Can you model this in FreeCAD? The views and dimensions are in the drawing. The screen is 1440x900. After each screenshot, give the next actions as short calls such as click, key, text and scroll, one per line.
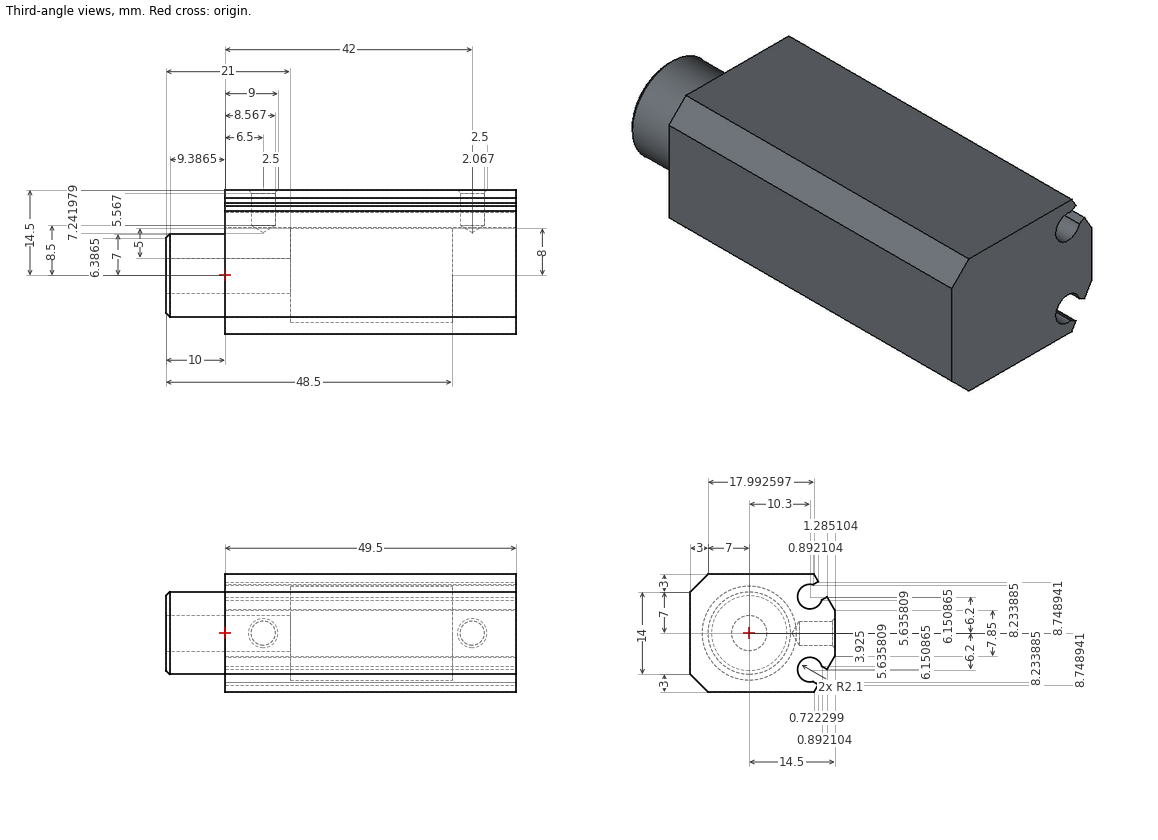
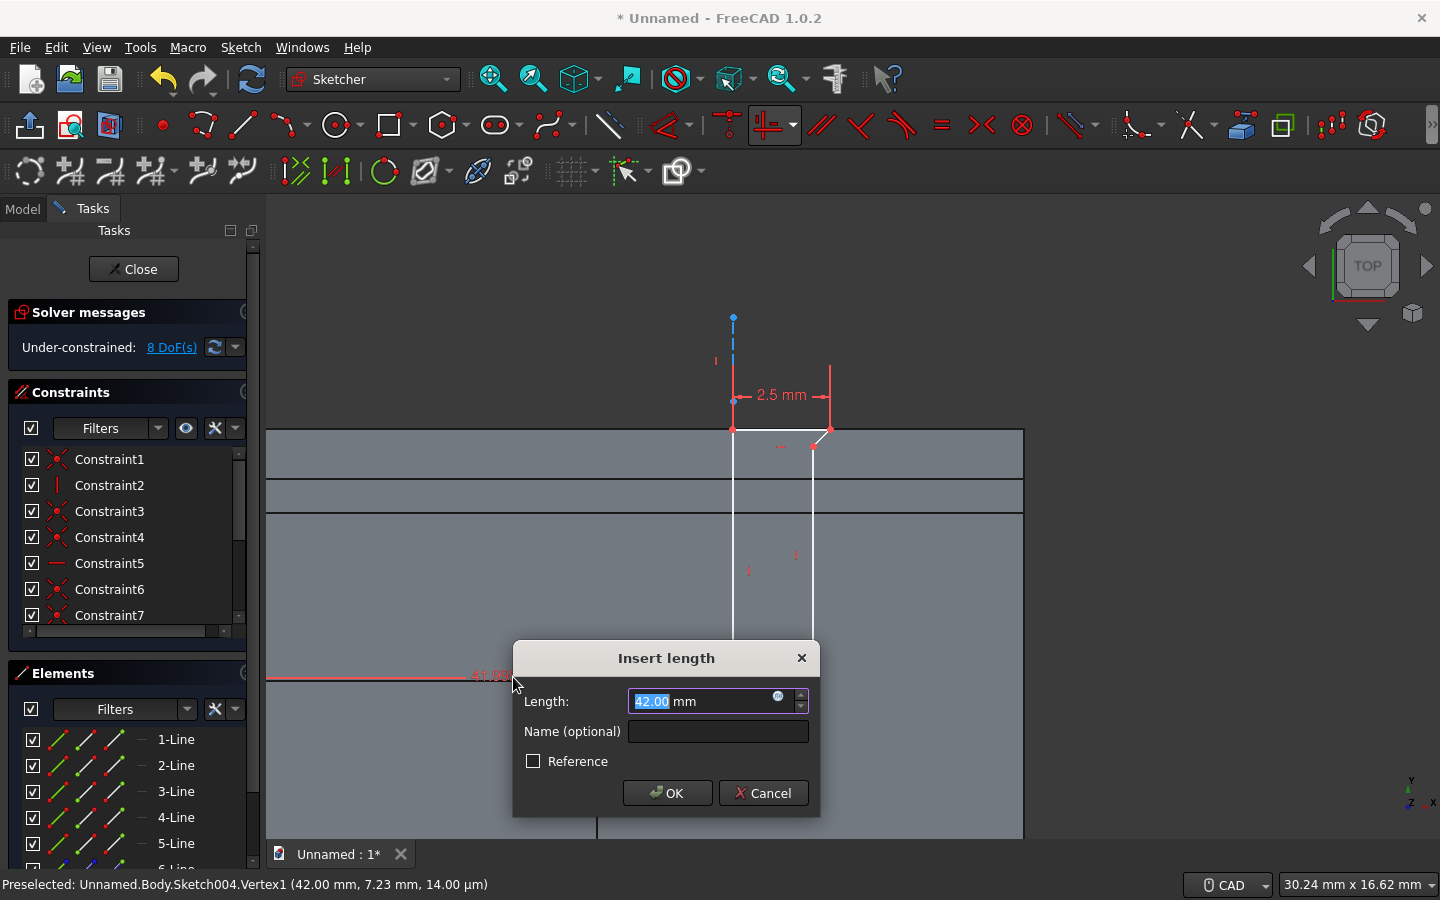
text(42)
key(Return)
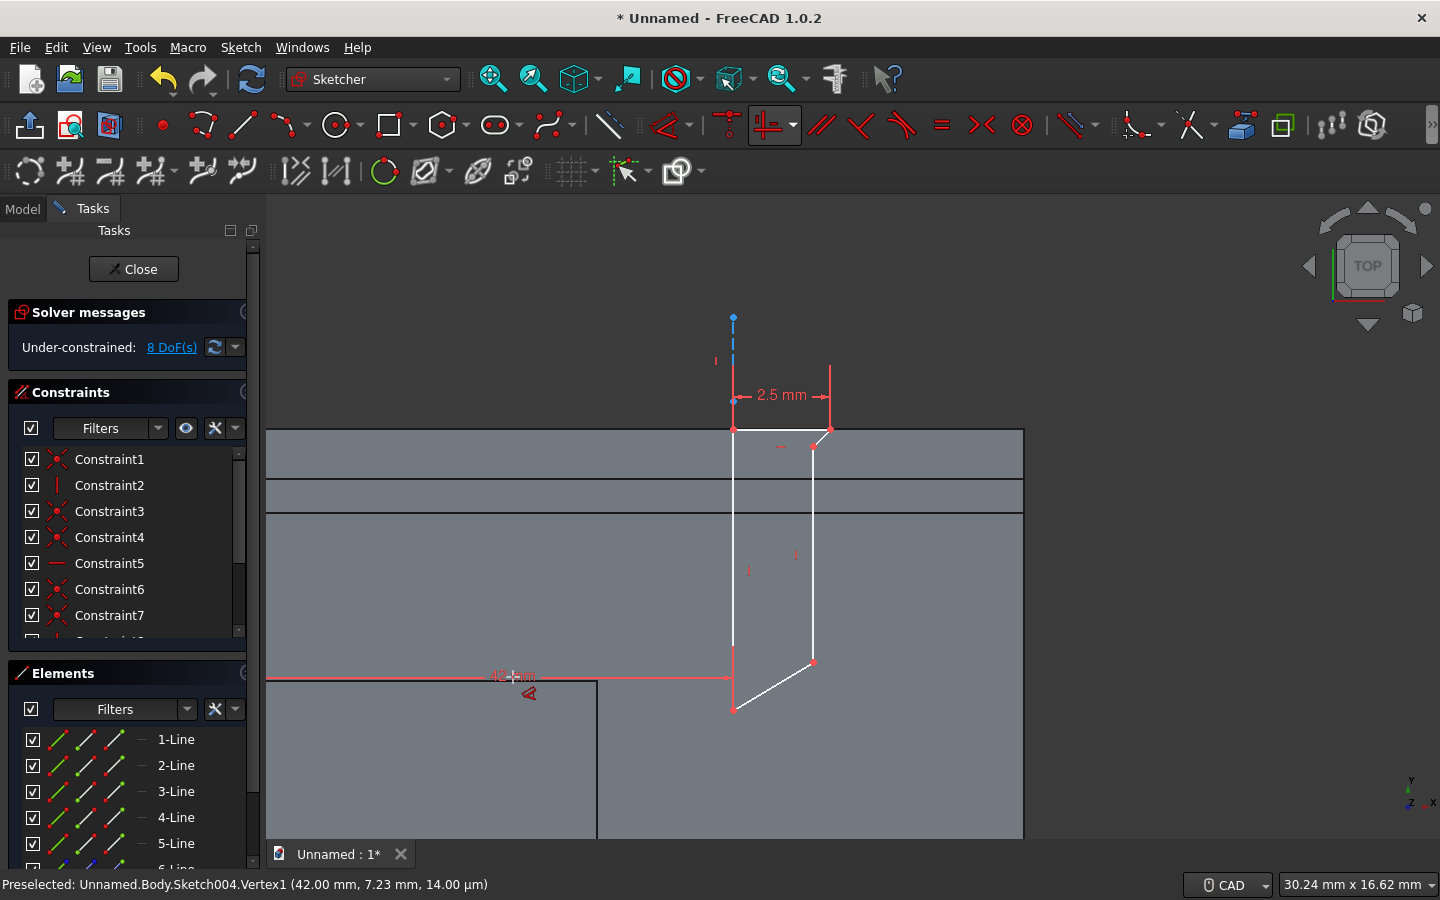
click(733, 402)
click(514, 368)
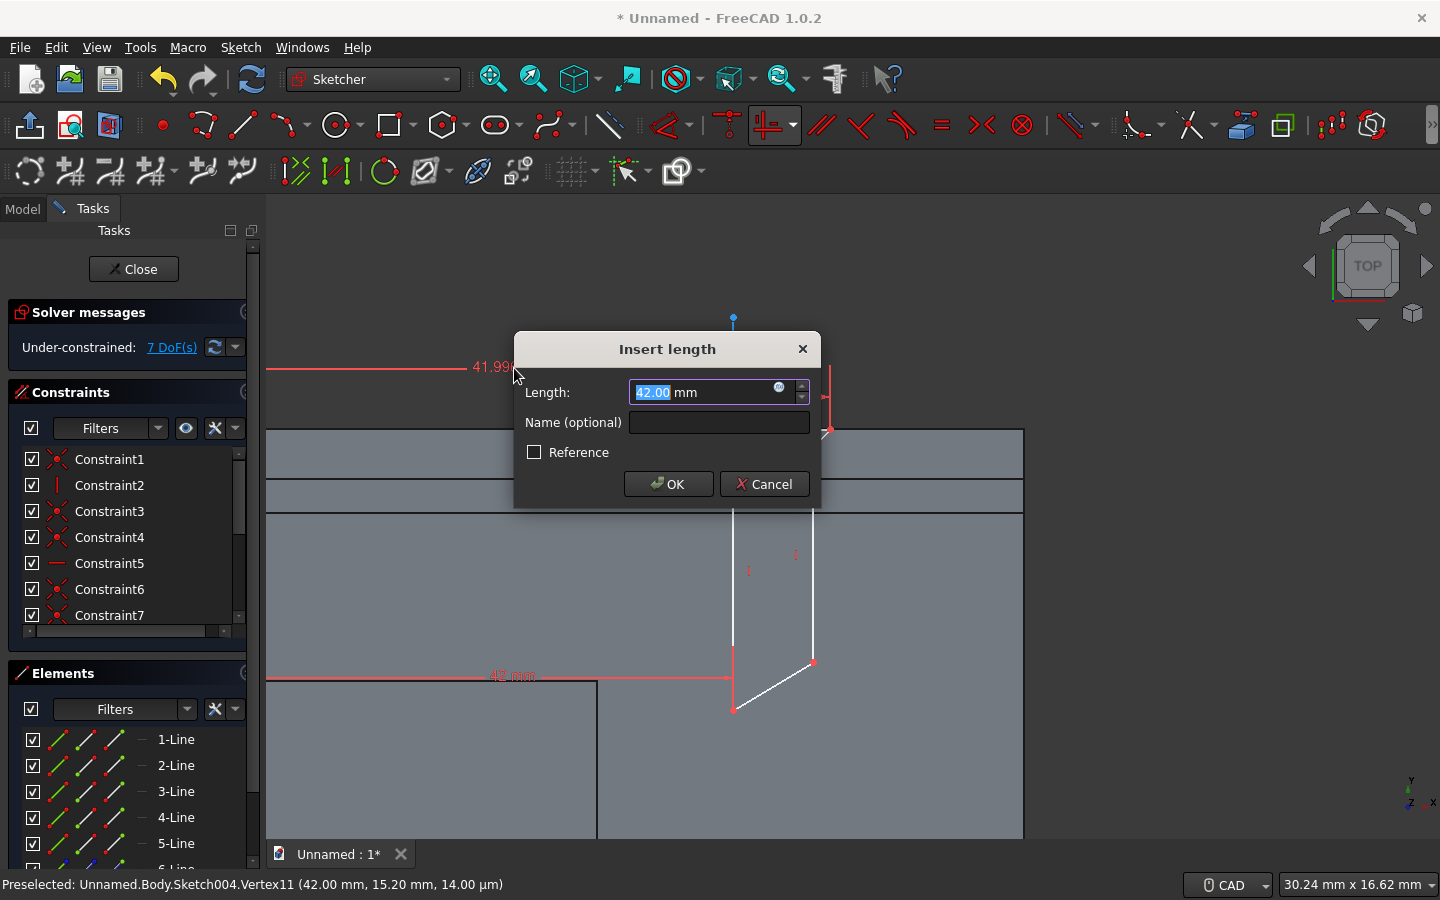
text(42)
key(Return)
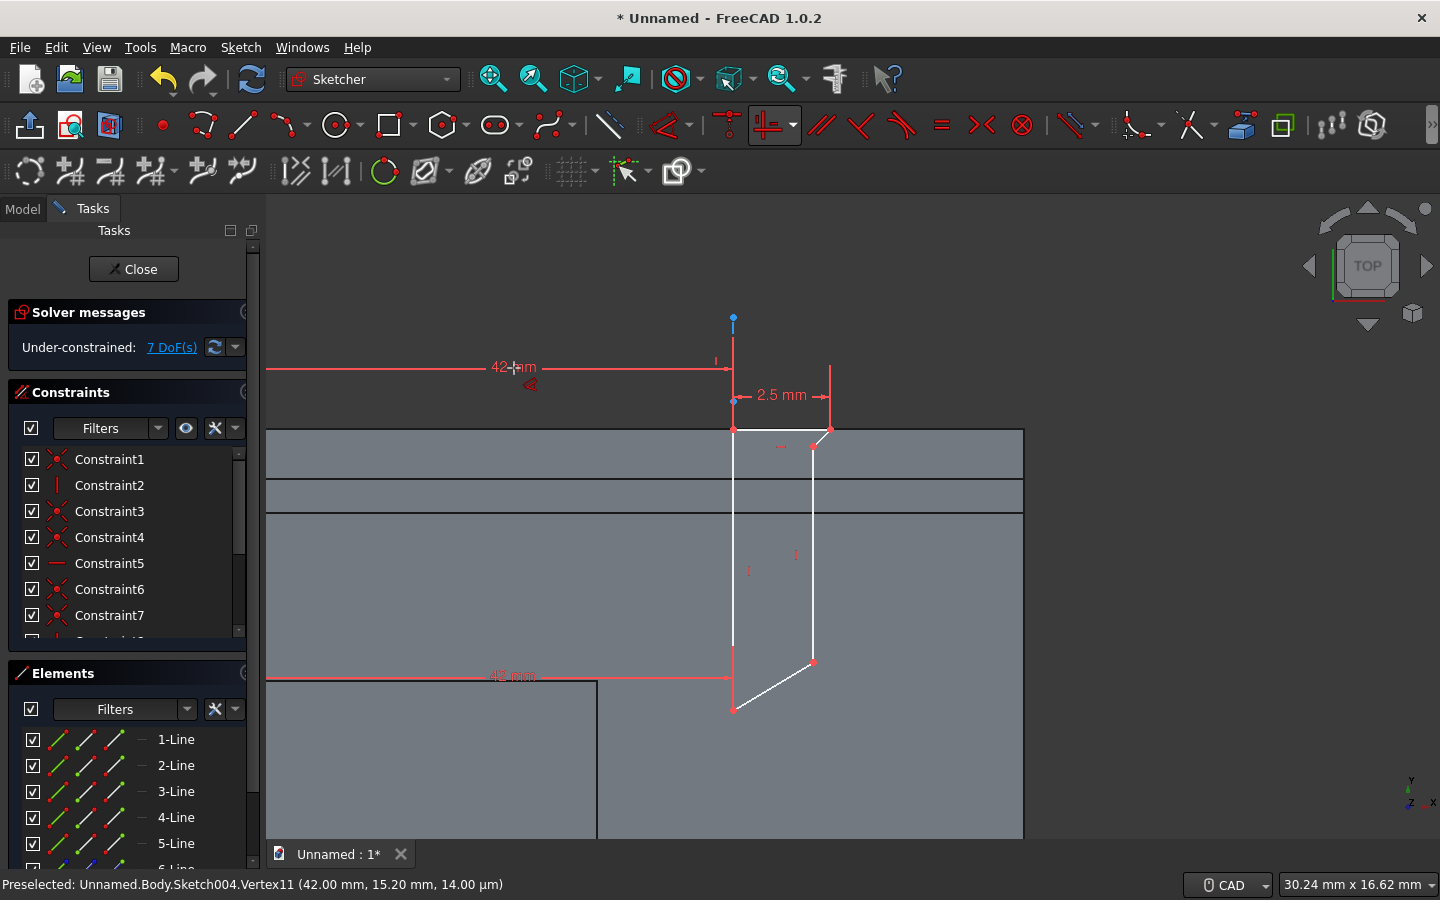
click(813, 663)
click(847, 737)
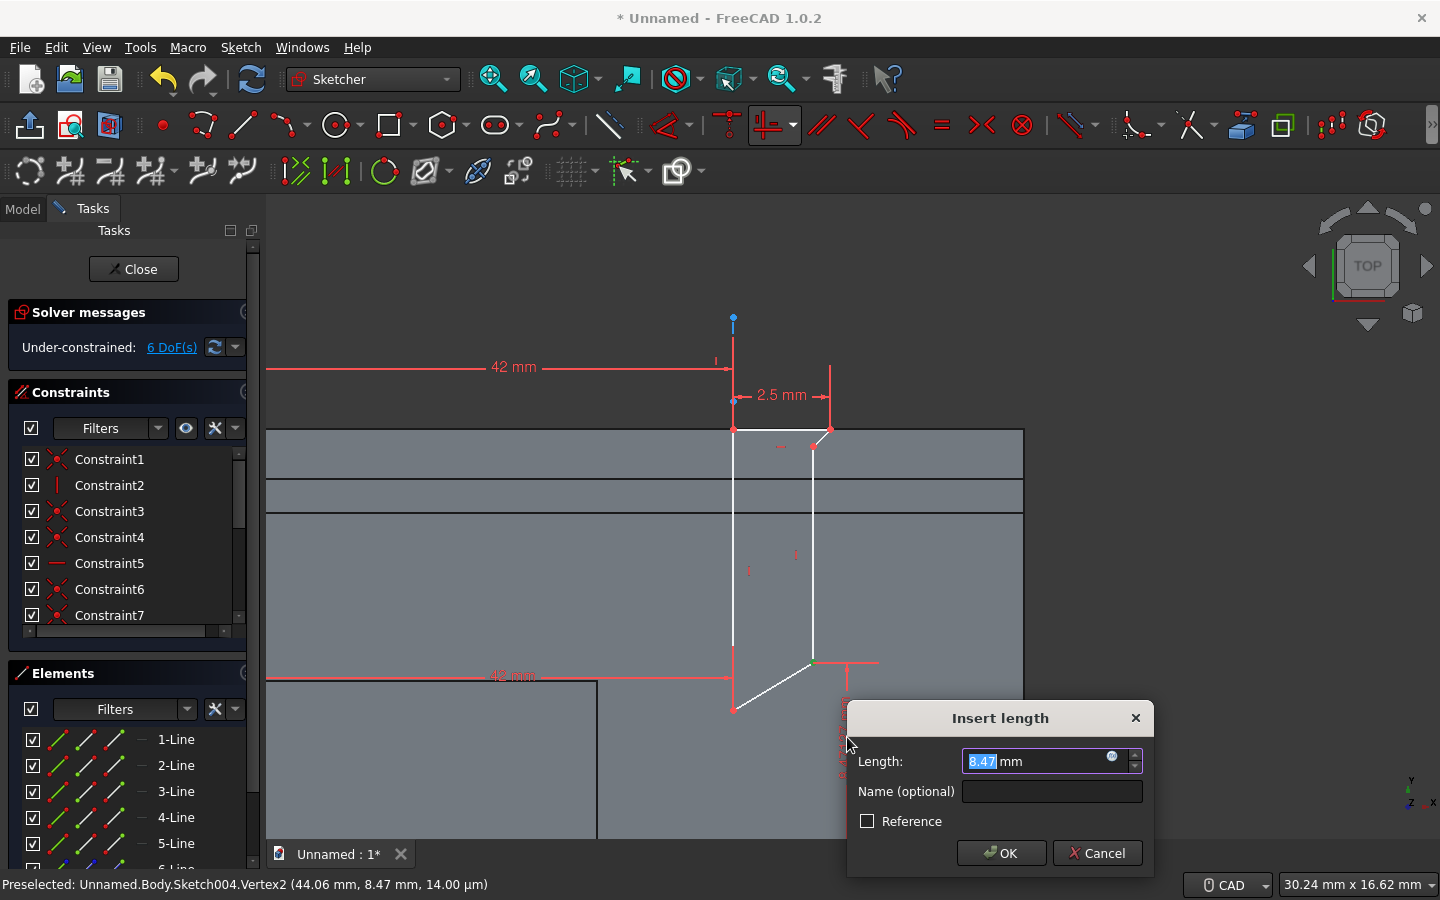
text(8.5)
key(Return)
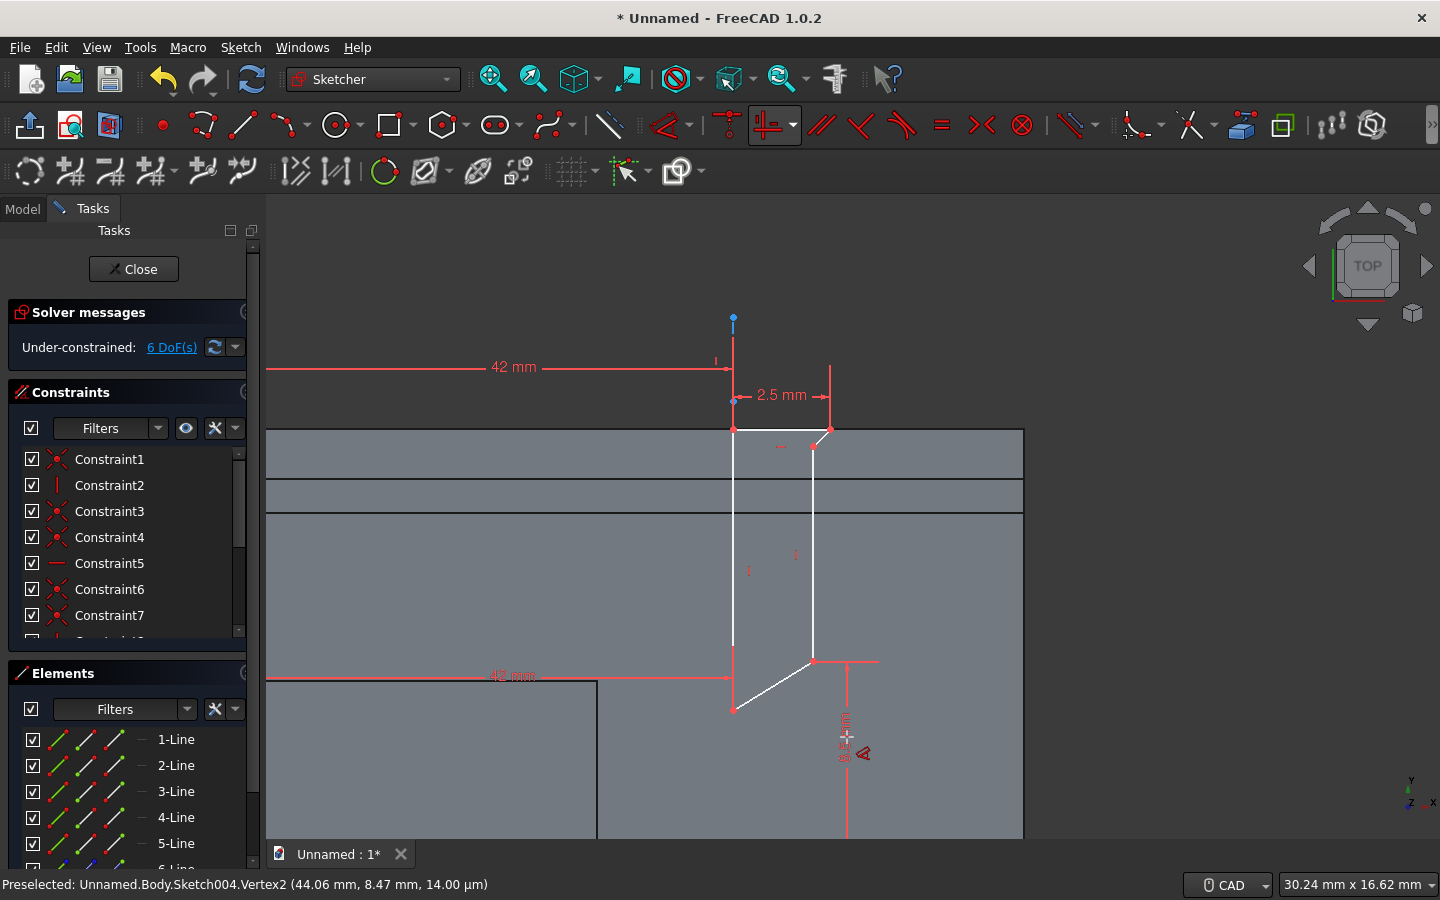
click(813, 597)
click(847, 554)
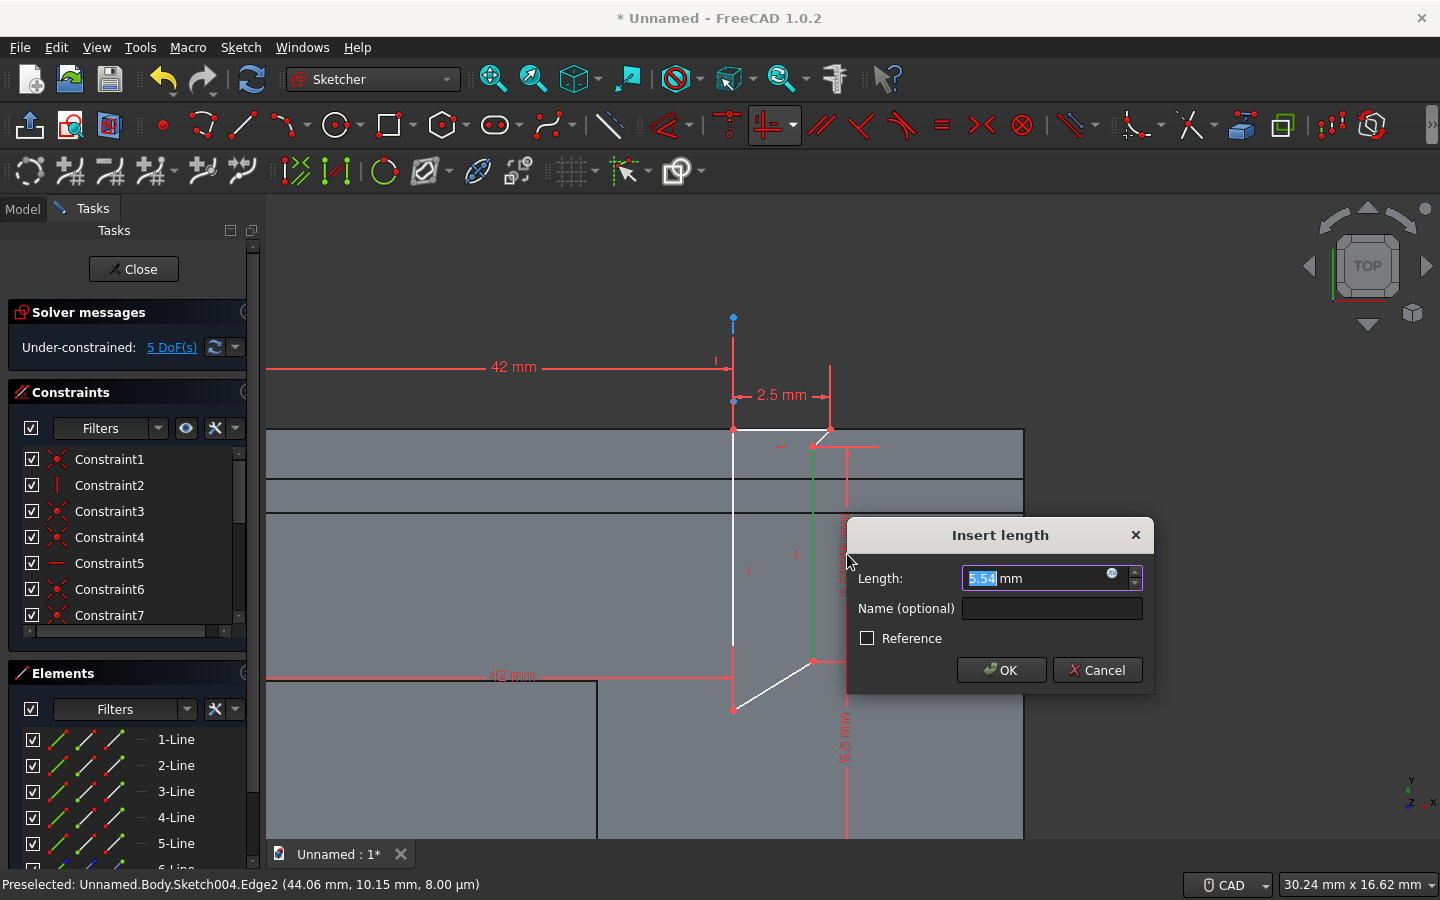
text(5.567)
key(Return)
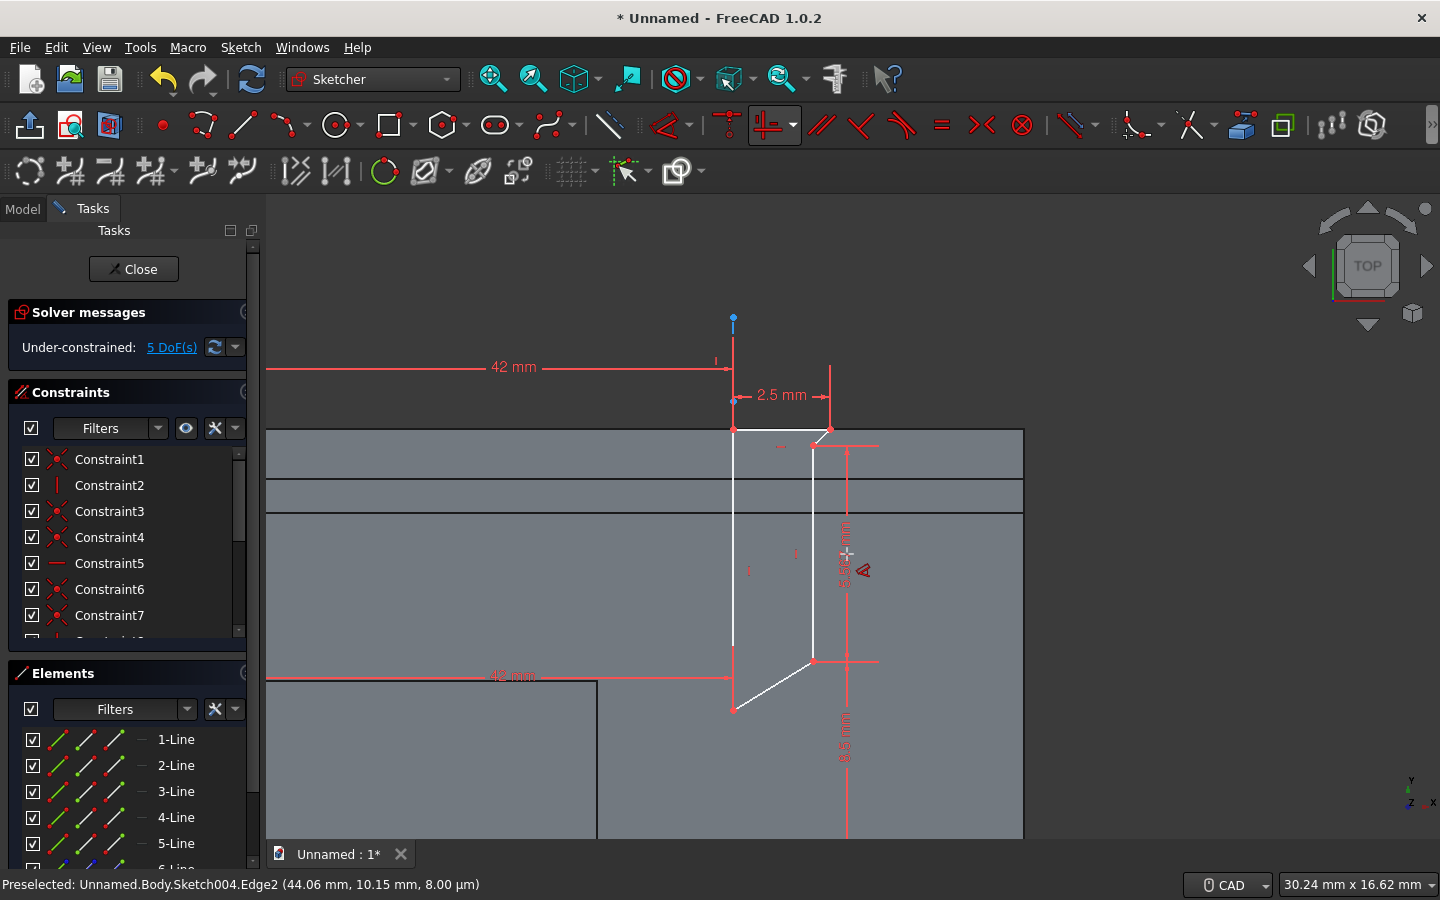
click(830, 430)
click(864, 621)